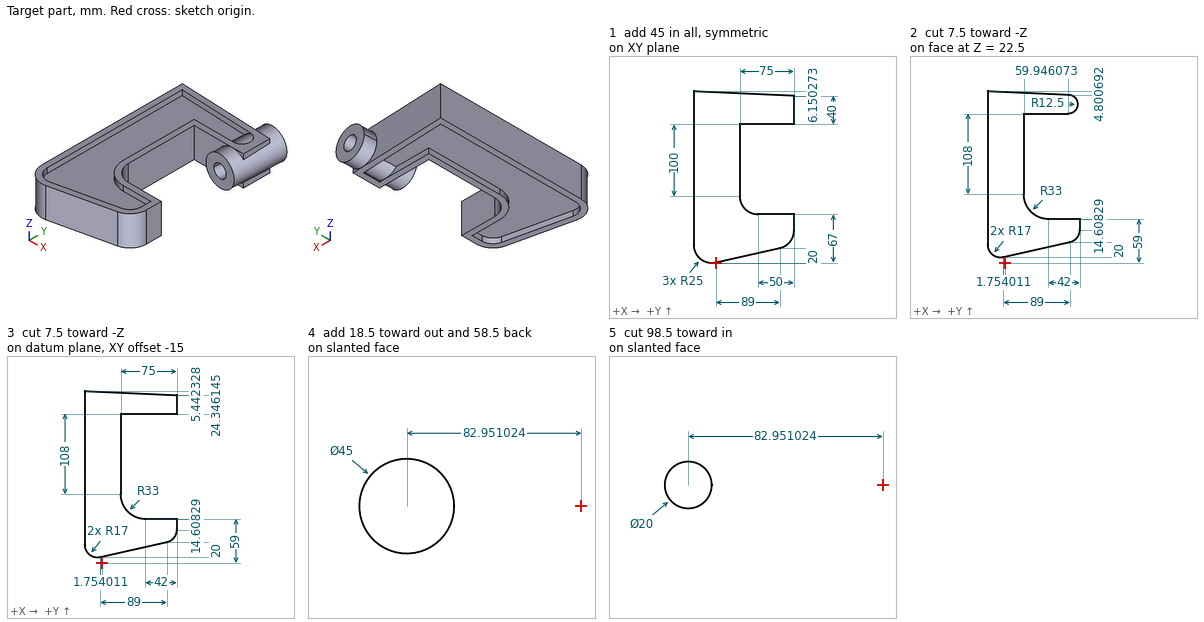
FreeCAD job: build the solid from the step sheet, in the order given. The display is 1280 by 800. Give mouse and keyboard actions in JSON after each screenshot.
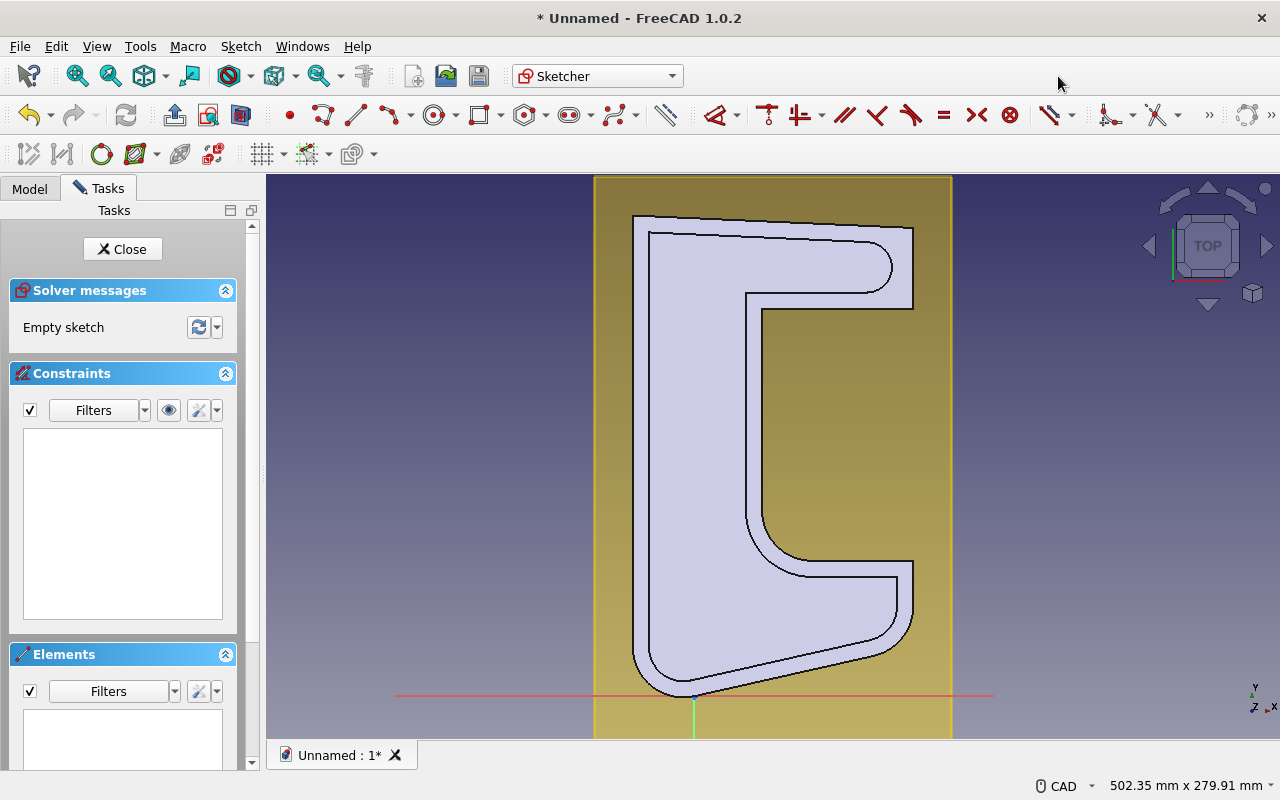
{"action": "left_click", "coordinate": [241, 116]}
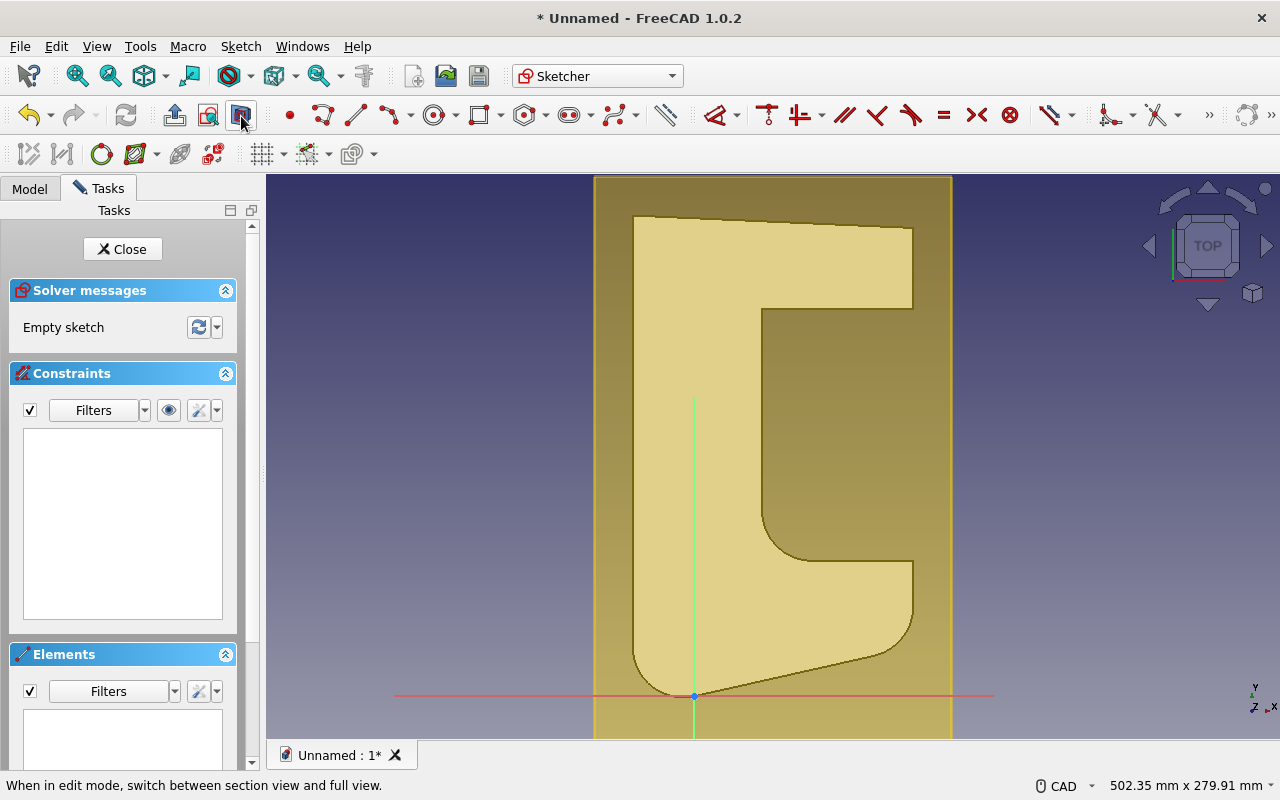
{"action": "scroll", "coordinate": [395, 421], "scroll_direction": "down", "scroll_amount": 1}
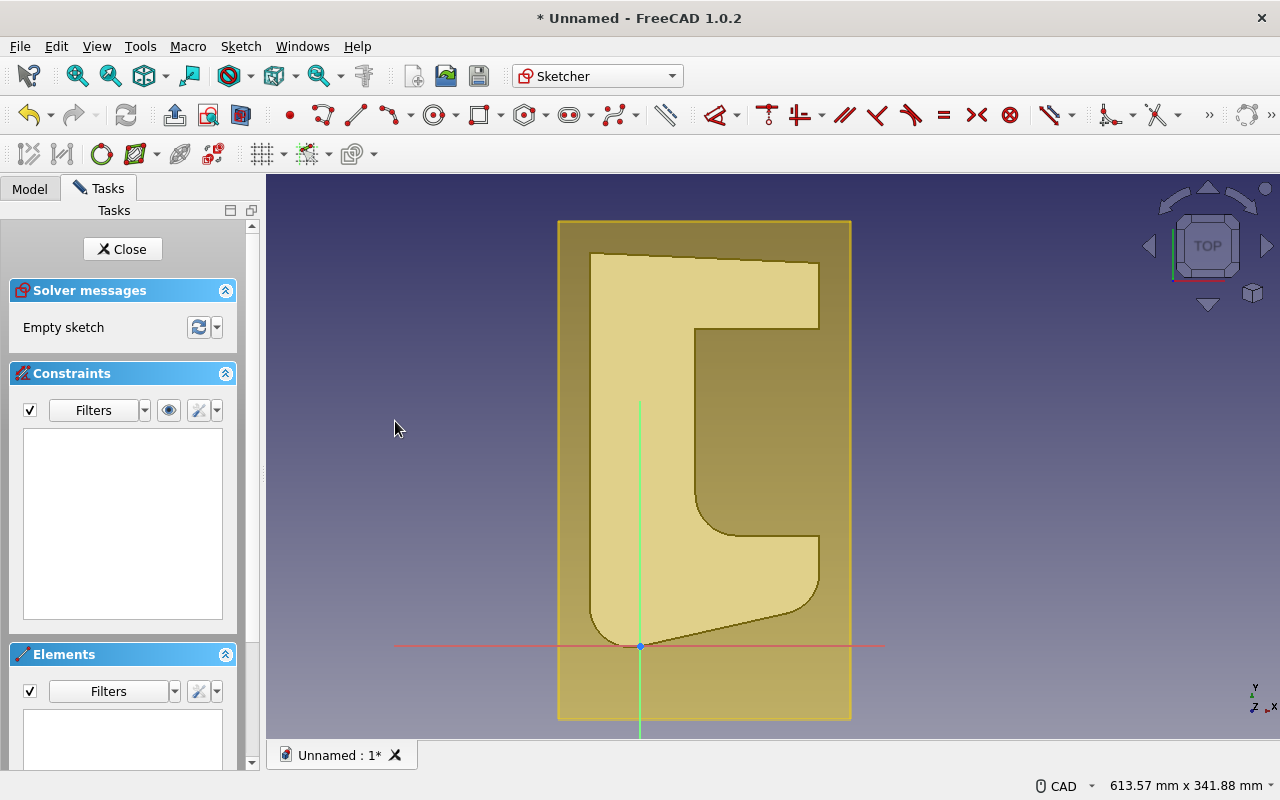
{"action": "left_click", "coordinate": [323, 116]}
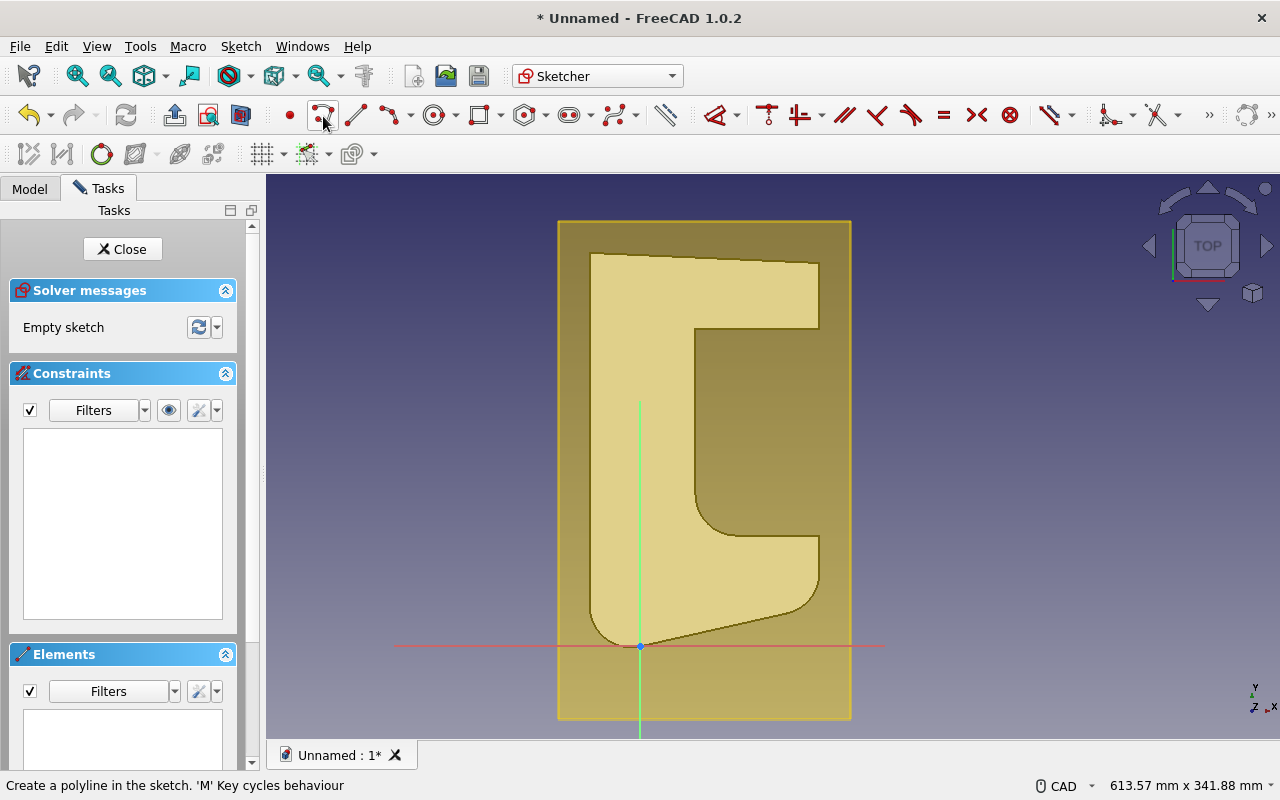
{"action": "left_click", "coordinate": [737, 549]}
{"action": "left_click", "coordinate": [806, 549]}
{"action": "left_click", "coordinate": [806, 573]}
{"action": "right_click", "coordinate": [806, 573]}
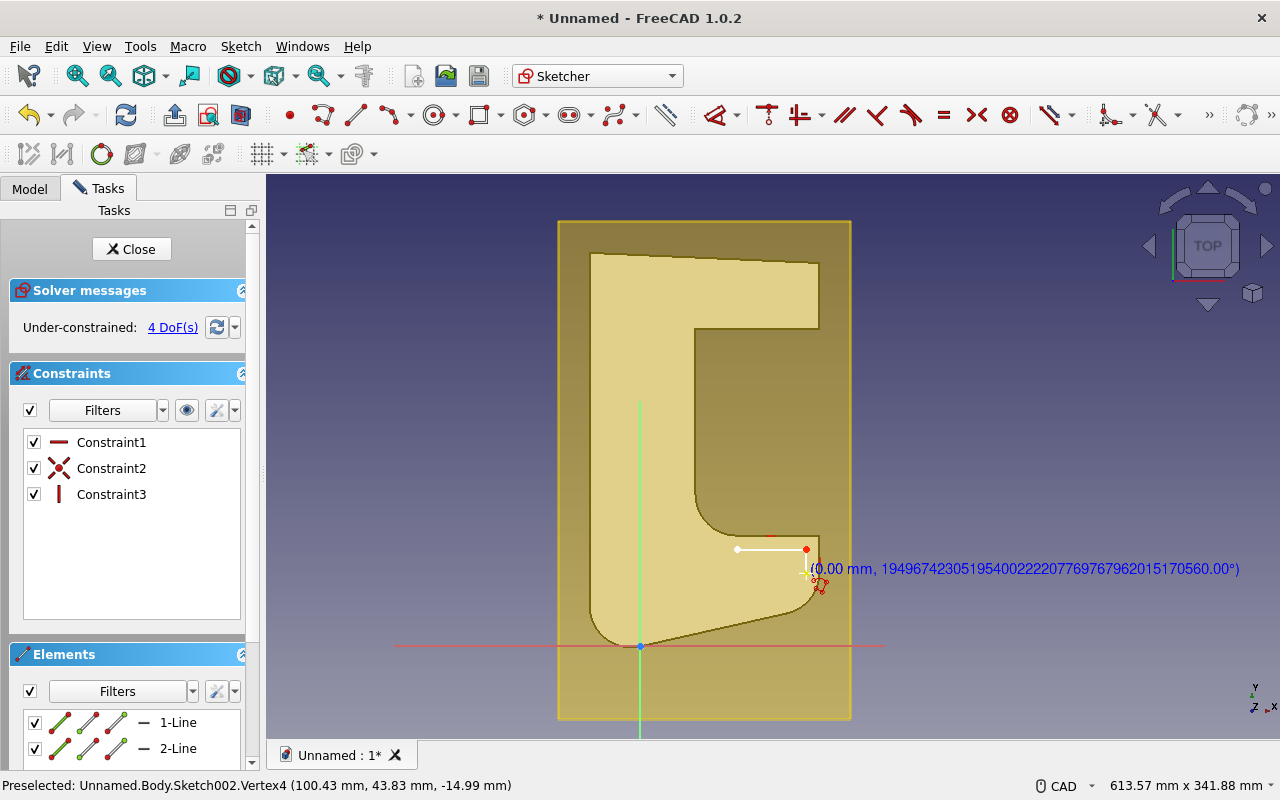
{"action": "left_click", "coordinate": [356, 116]}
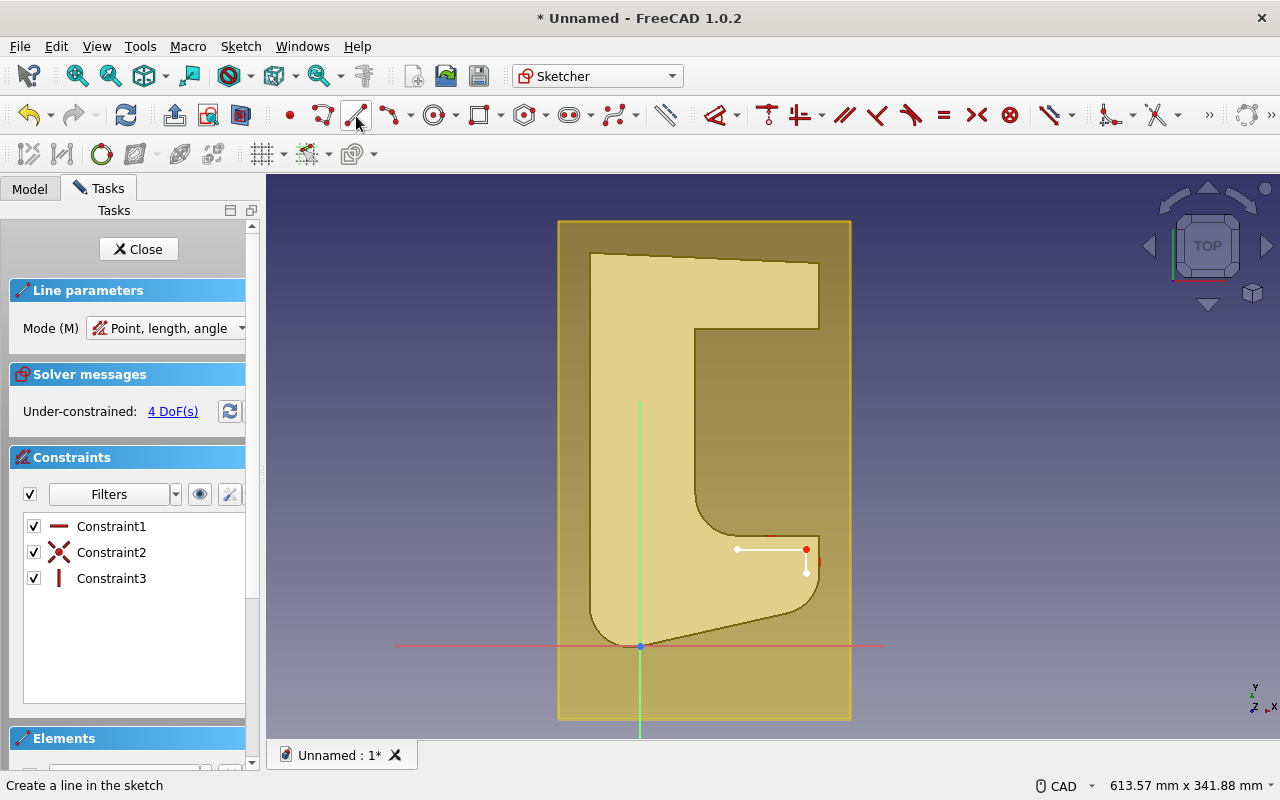
{"action": "left_click", "coordinate": [784, 600]}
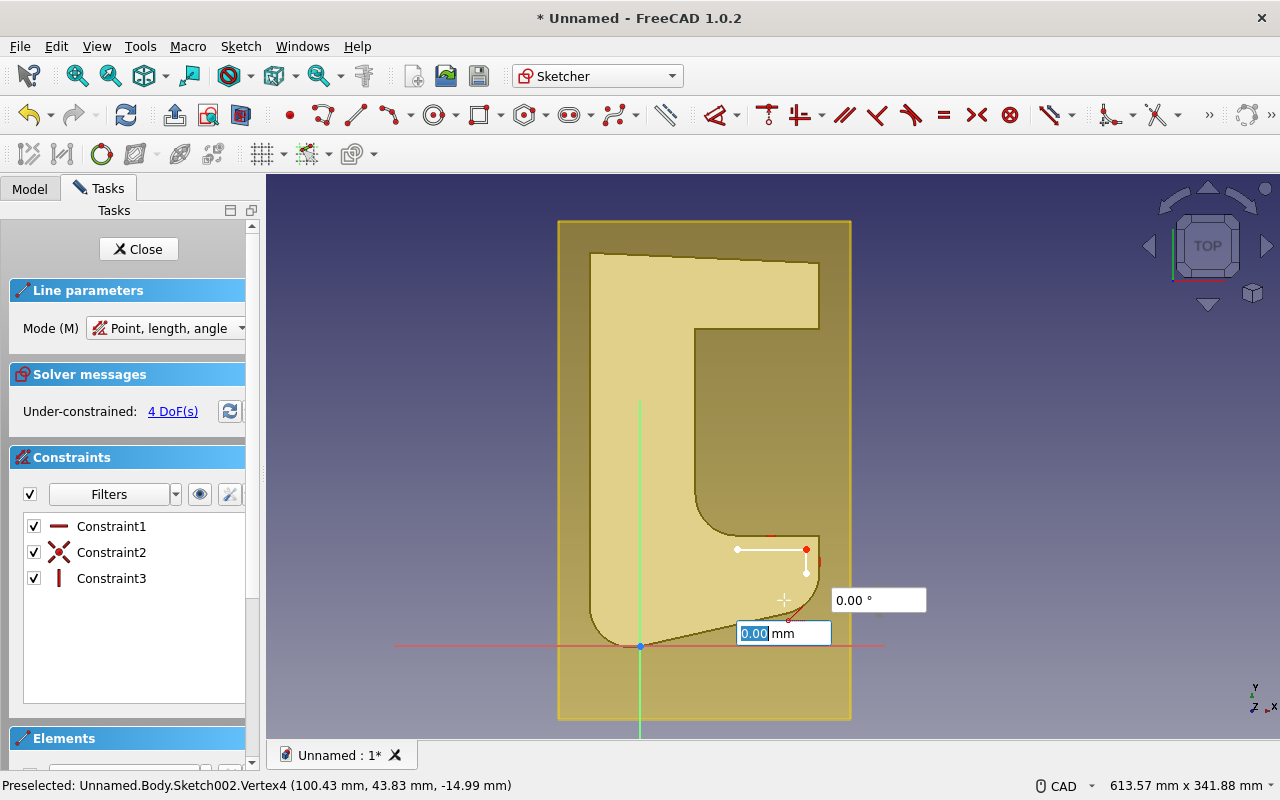
{"action": "scroll", "coordinate": [637, 634], "scroll_direction": "up", "scroll_amount": 9}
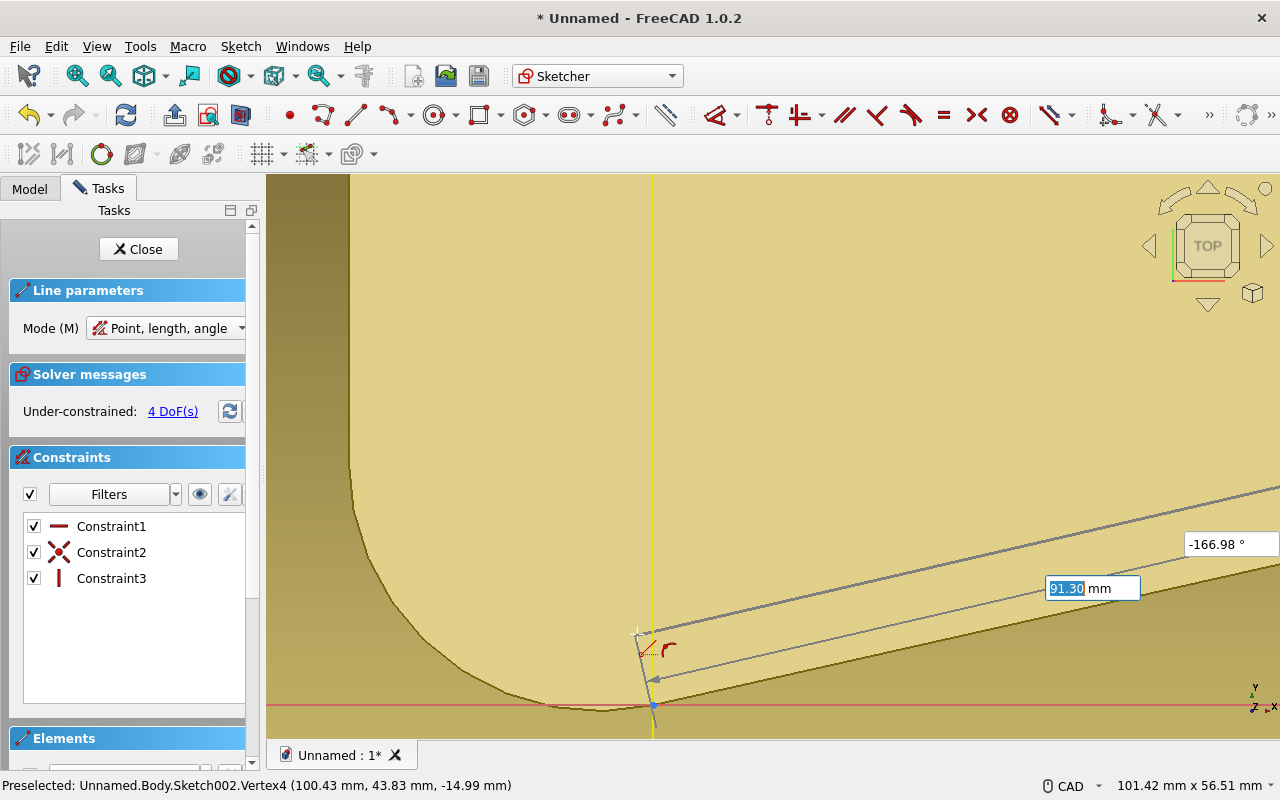
{"action": "left_click", "coordinate": [636, 627]}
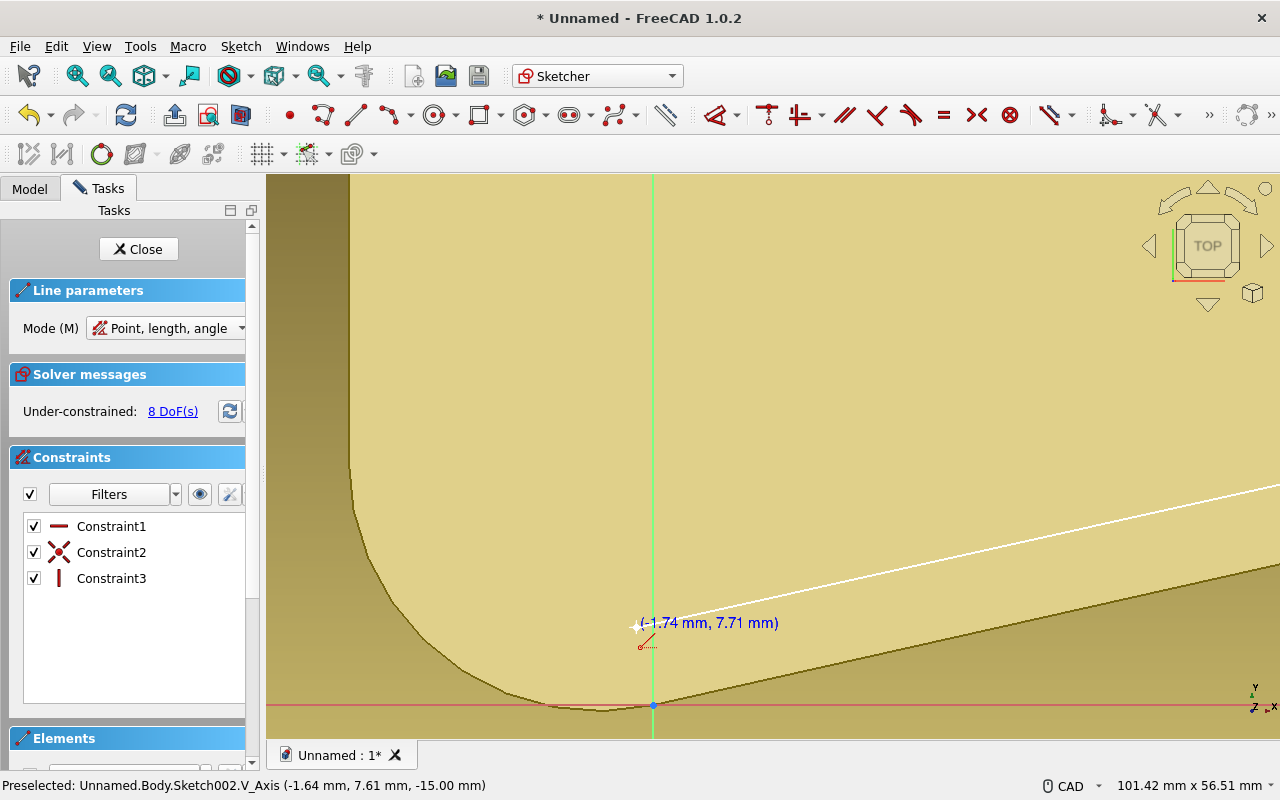
{"action": "left_click", "coordinate": [323, 116]}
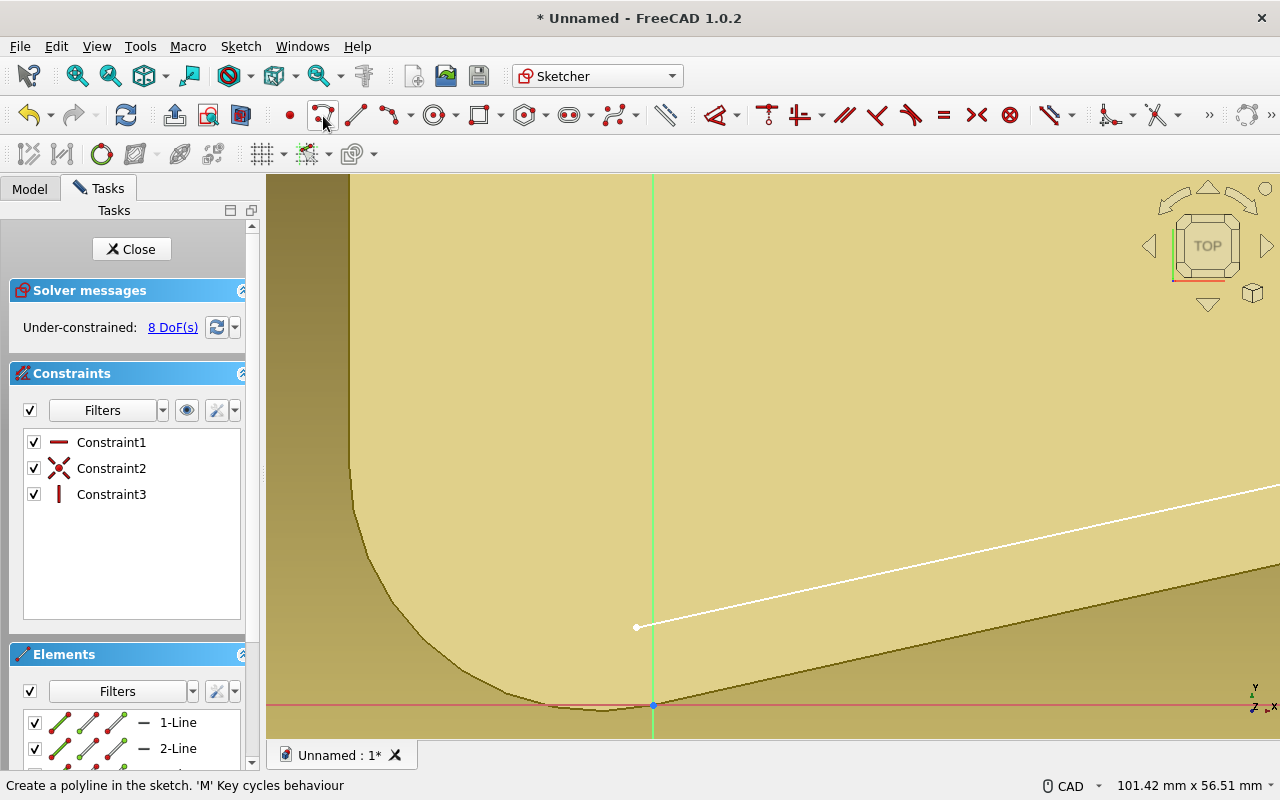
{"action": "scroll", "coordinate": [637, 635], "scroll_direction": "down", "scroll_amount": 9}